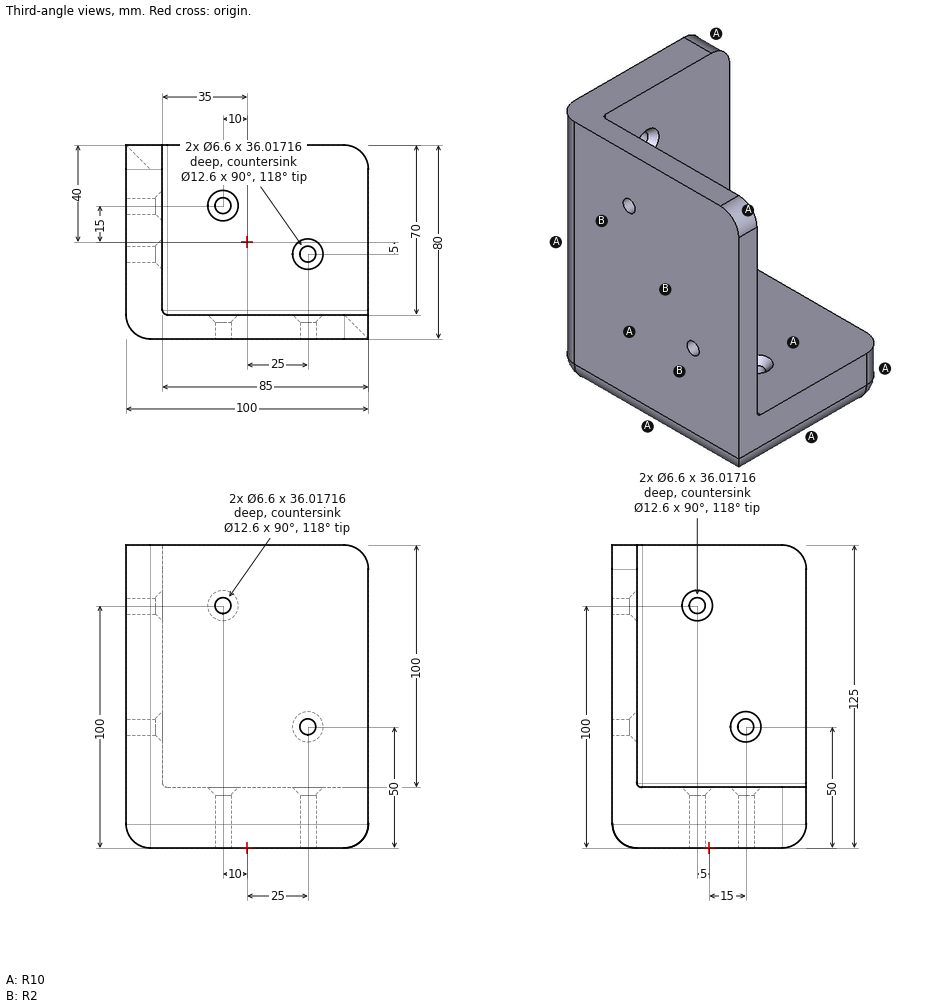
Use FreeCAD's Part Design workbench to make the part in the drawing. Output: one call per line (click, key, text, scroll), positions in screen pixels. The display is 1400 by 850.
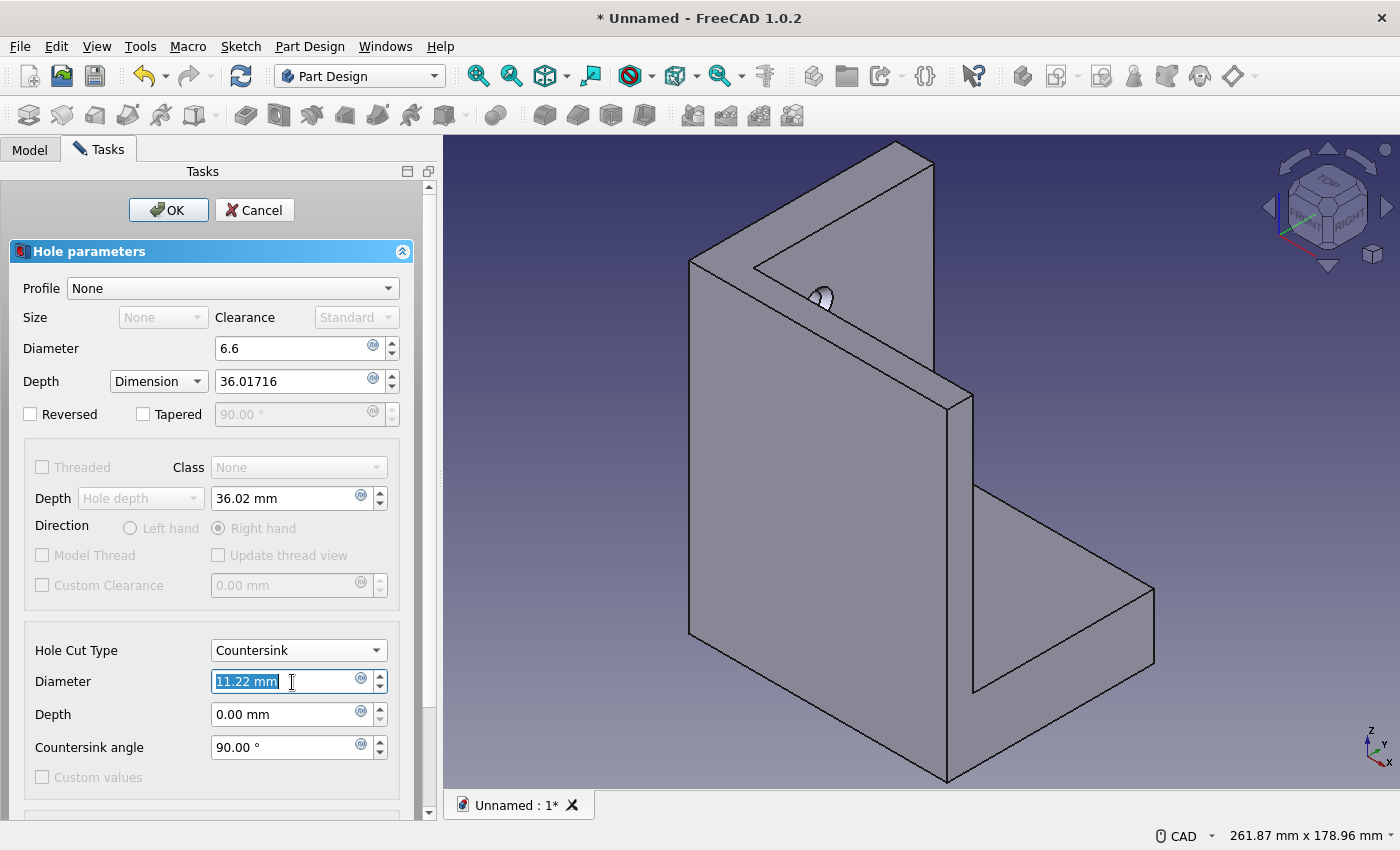
text(12.6)
key(Tab)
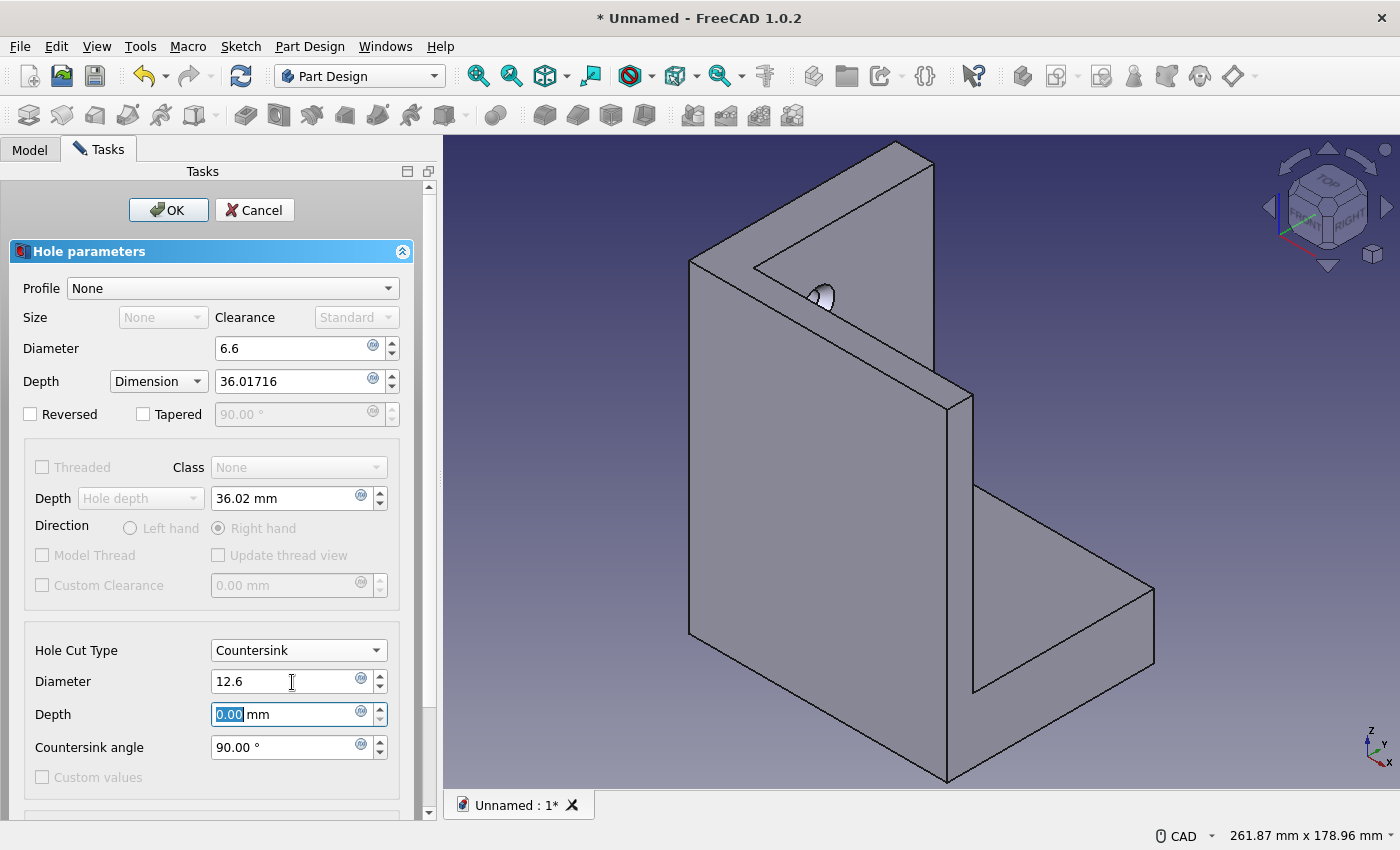
click(169, 210)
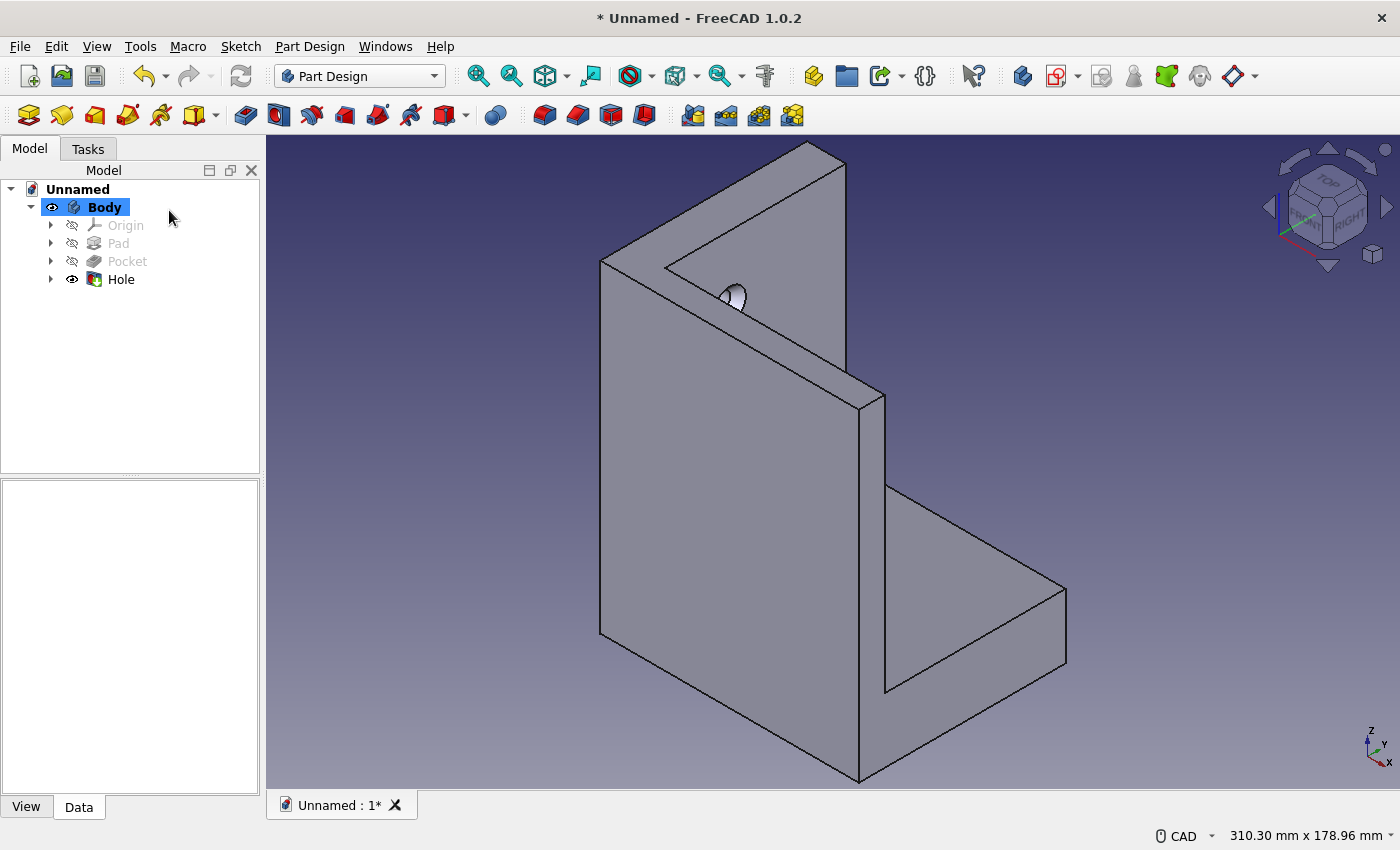
key(4)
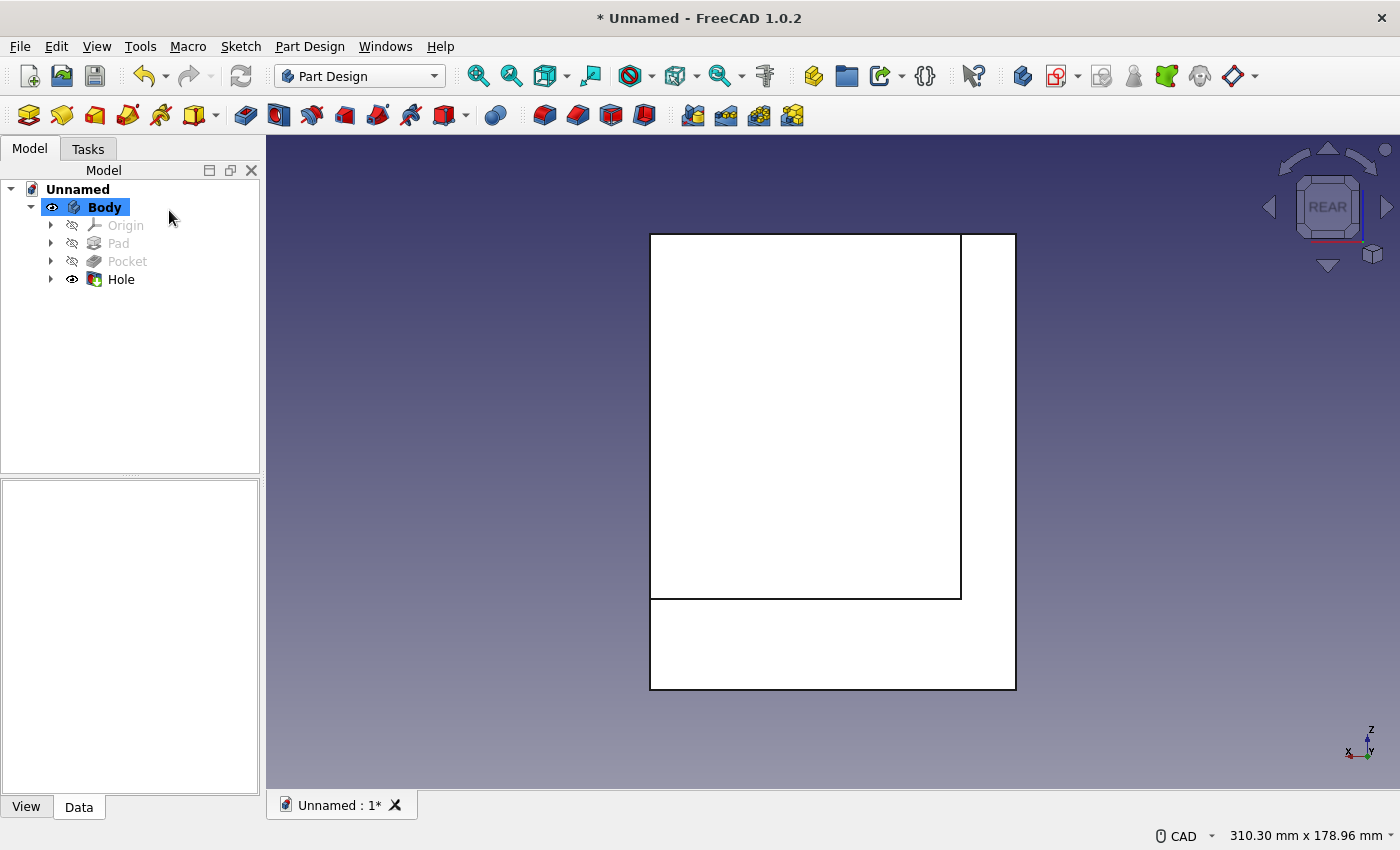
click(806, 415)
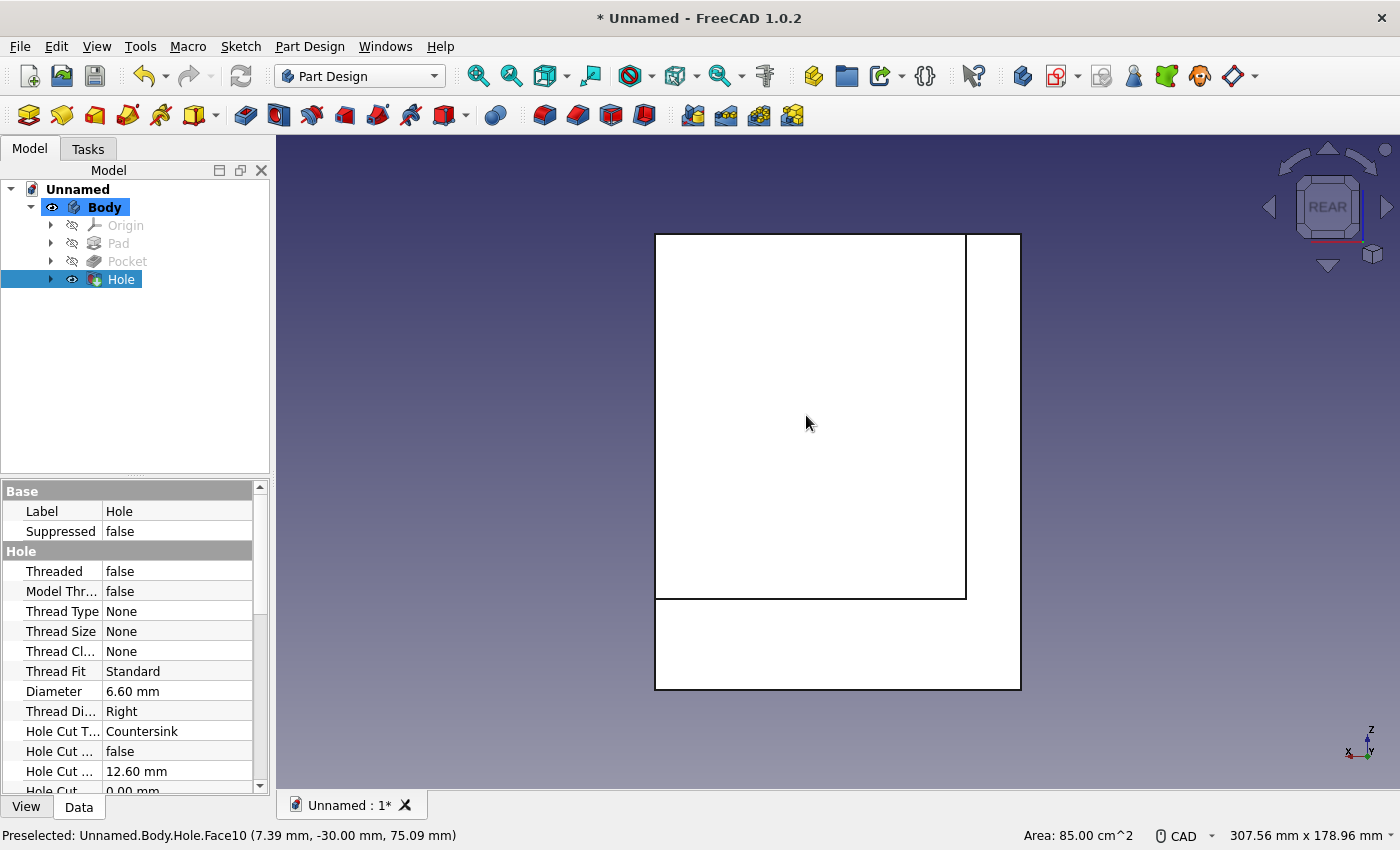
click(1056, 76)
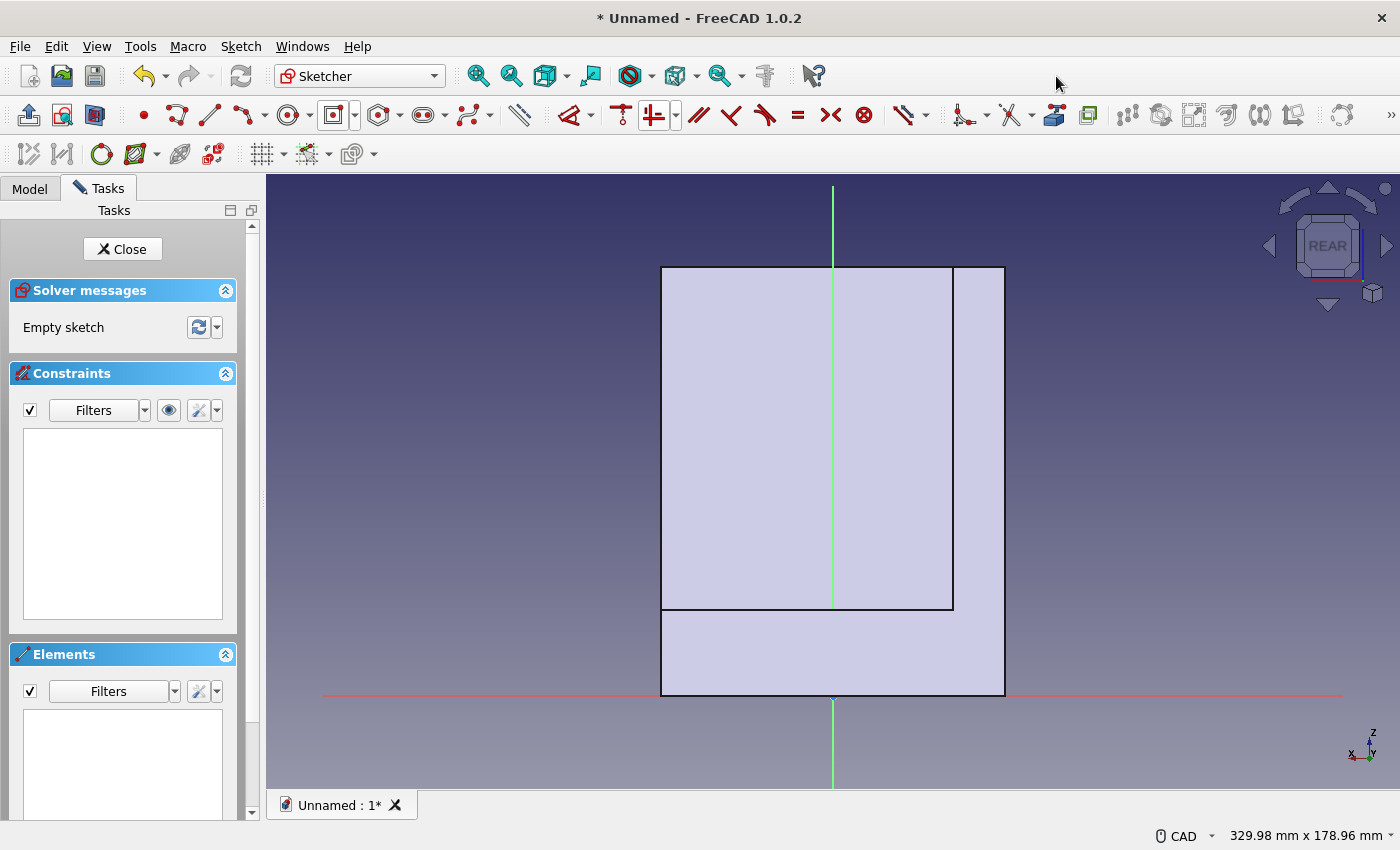
key(g)
key(c)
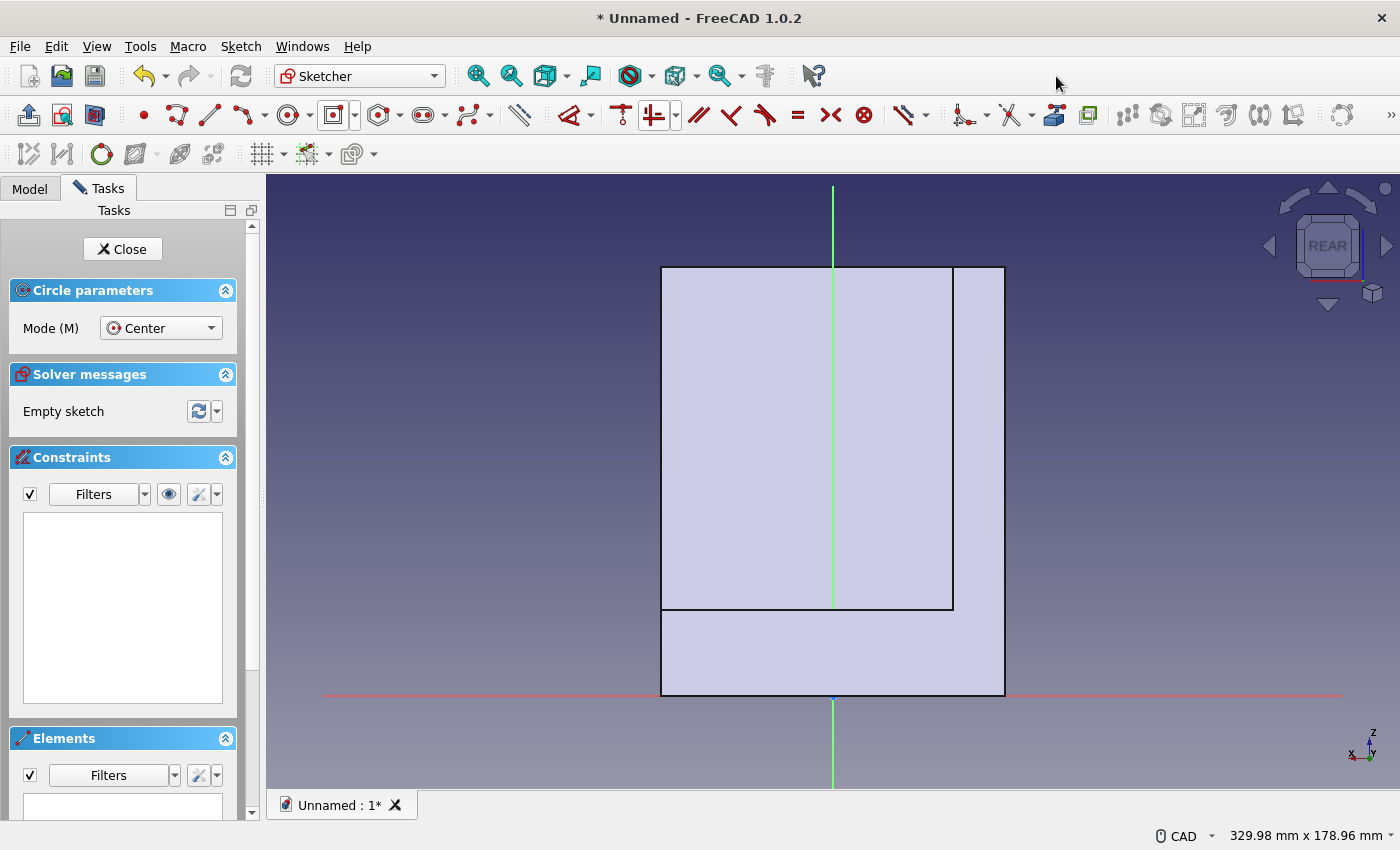
scroll(867, 353, up, 4)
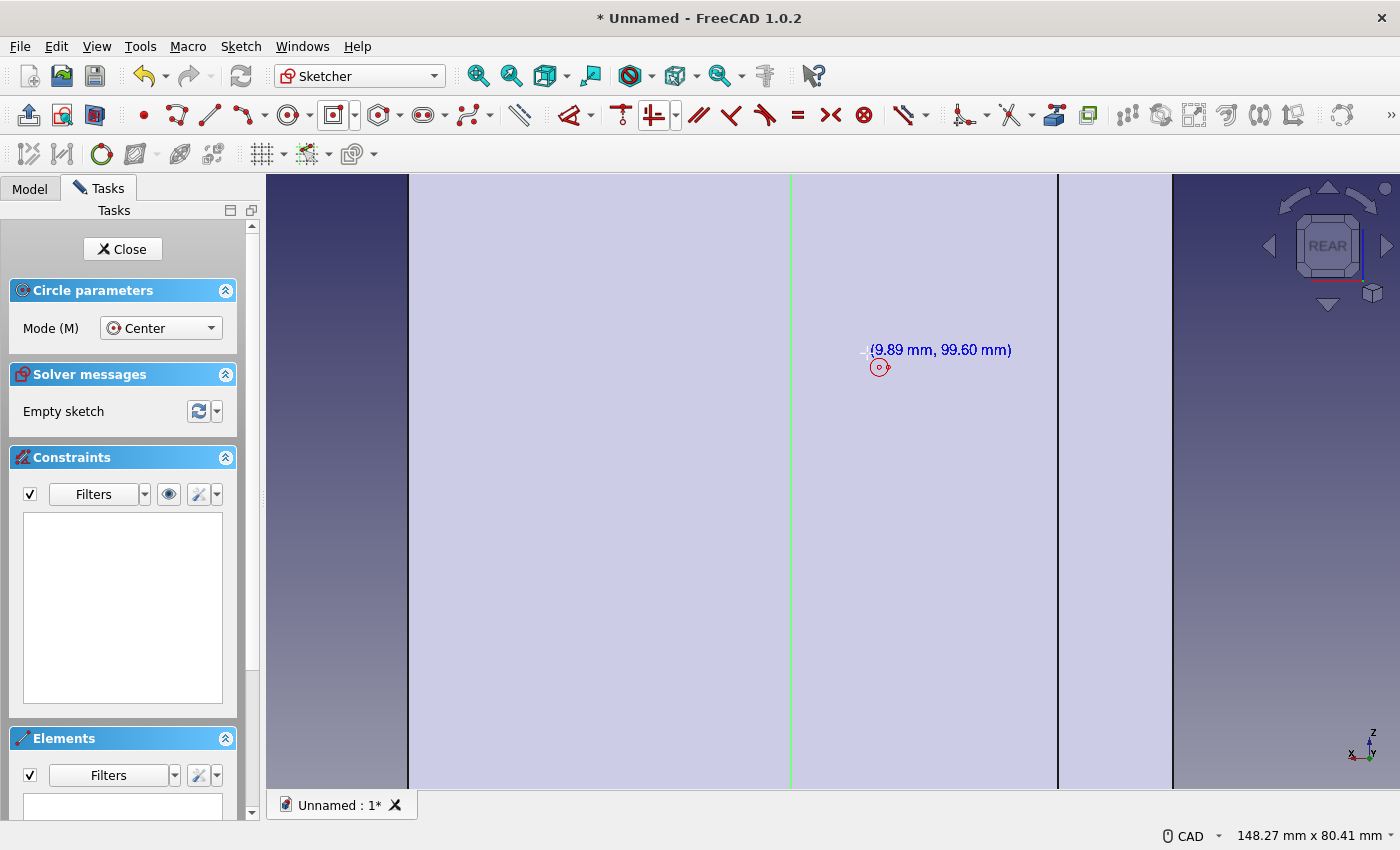
click(867, 352)
move(885, 334)